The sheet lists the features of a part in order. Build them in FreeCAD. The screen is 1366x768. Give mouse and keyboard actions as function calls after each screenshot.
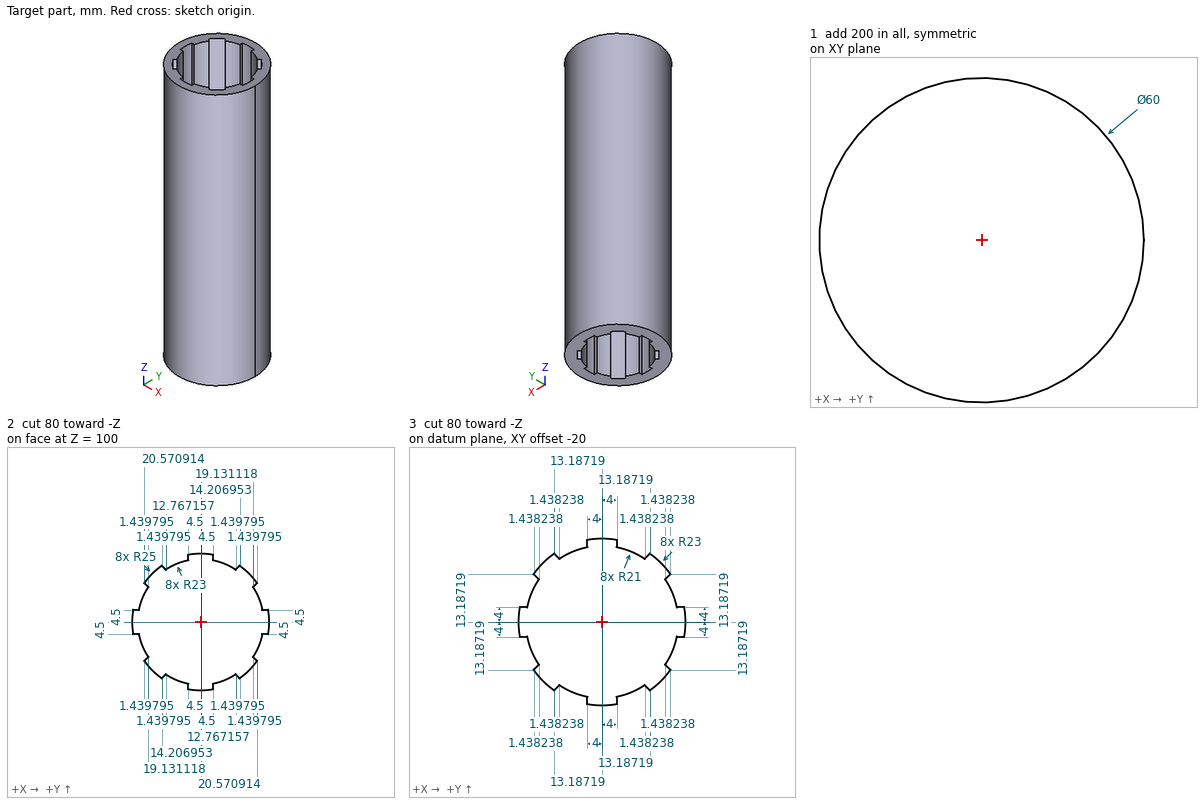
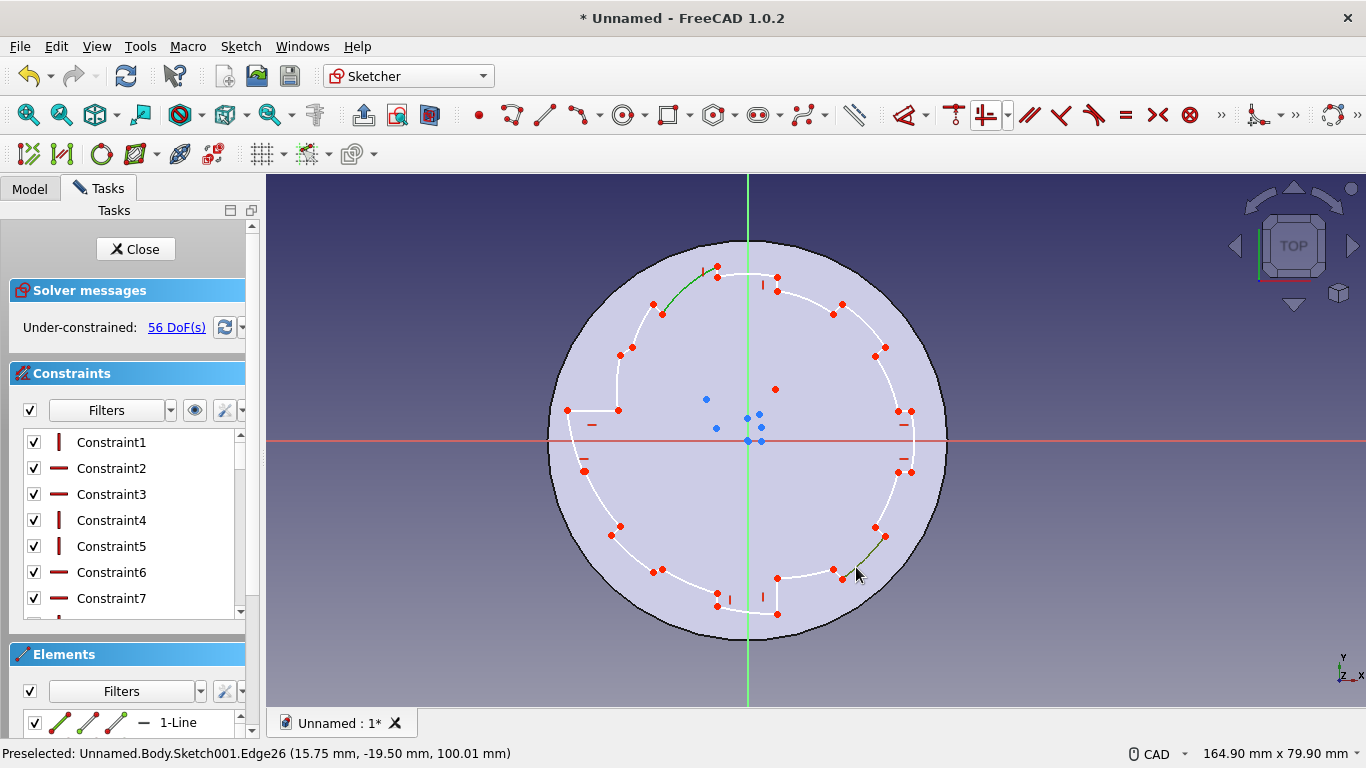
click(954, 116)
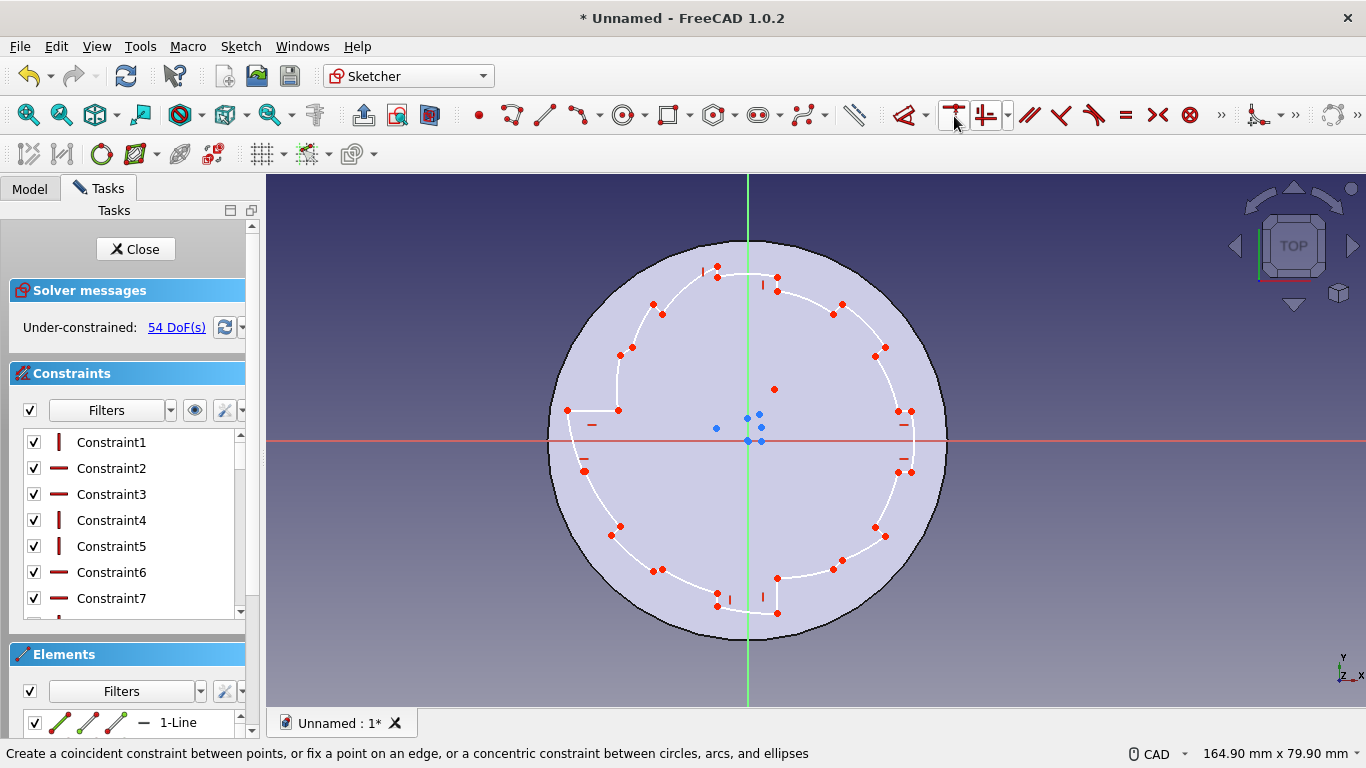
click(698, 278)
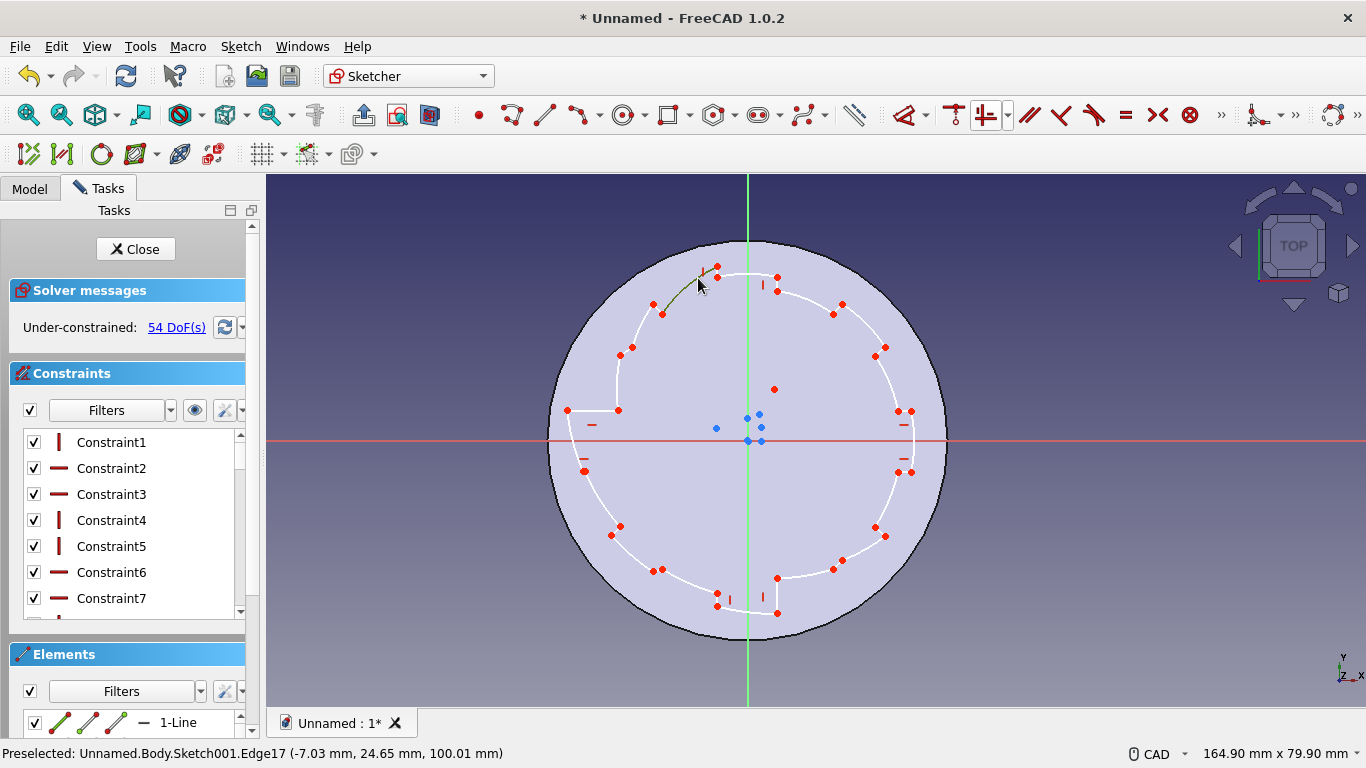
click(884, 511)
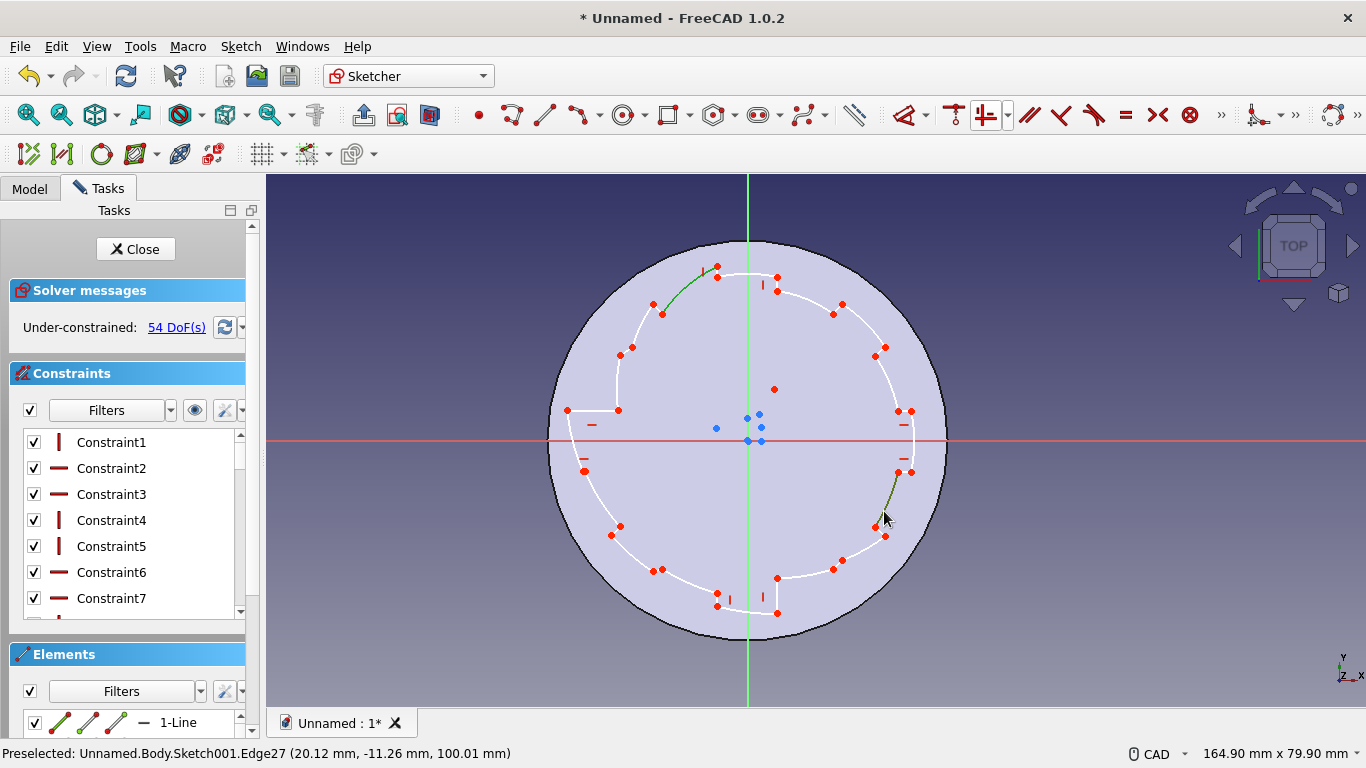
click(954, 116)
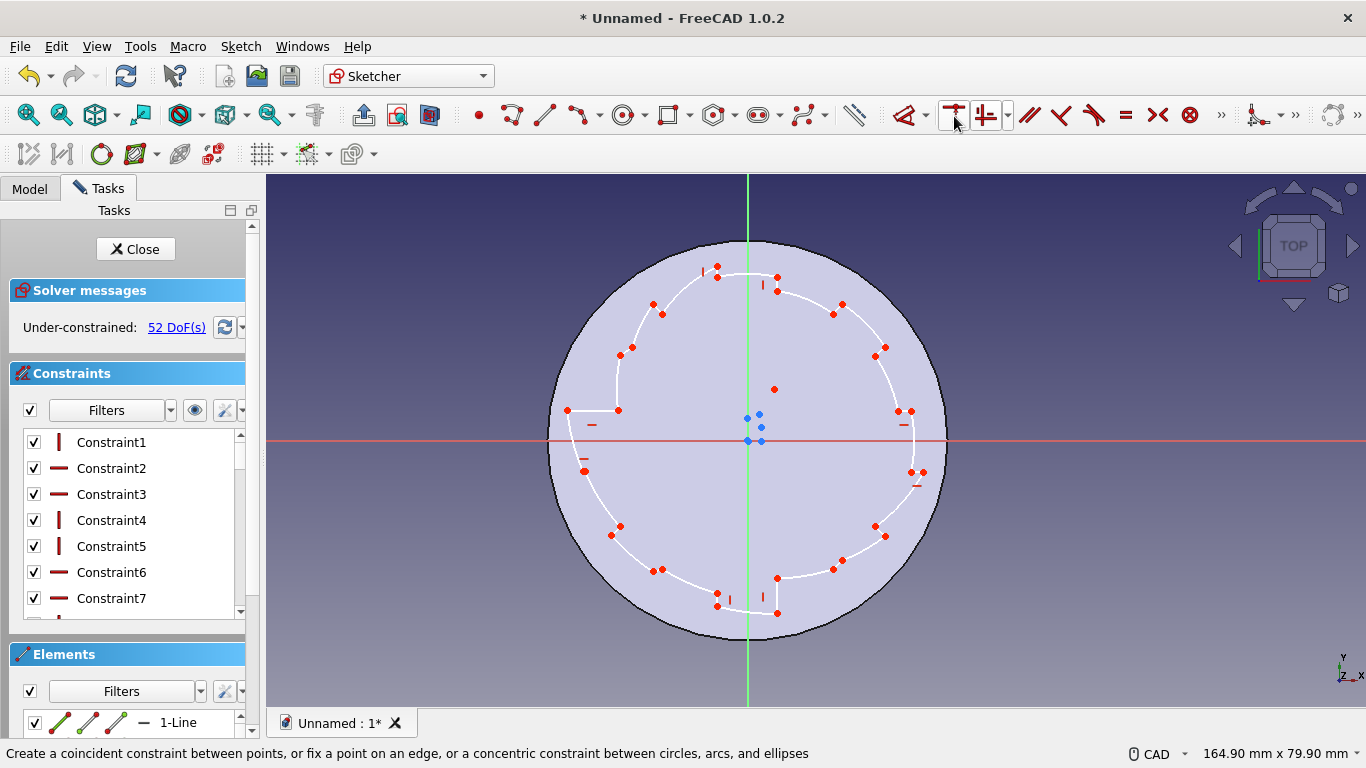
click(698, 278)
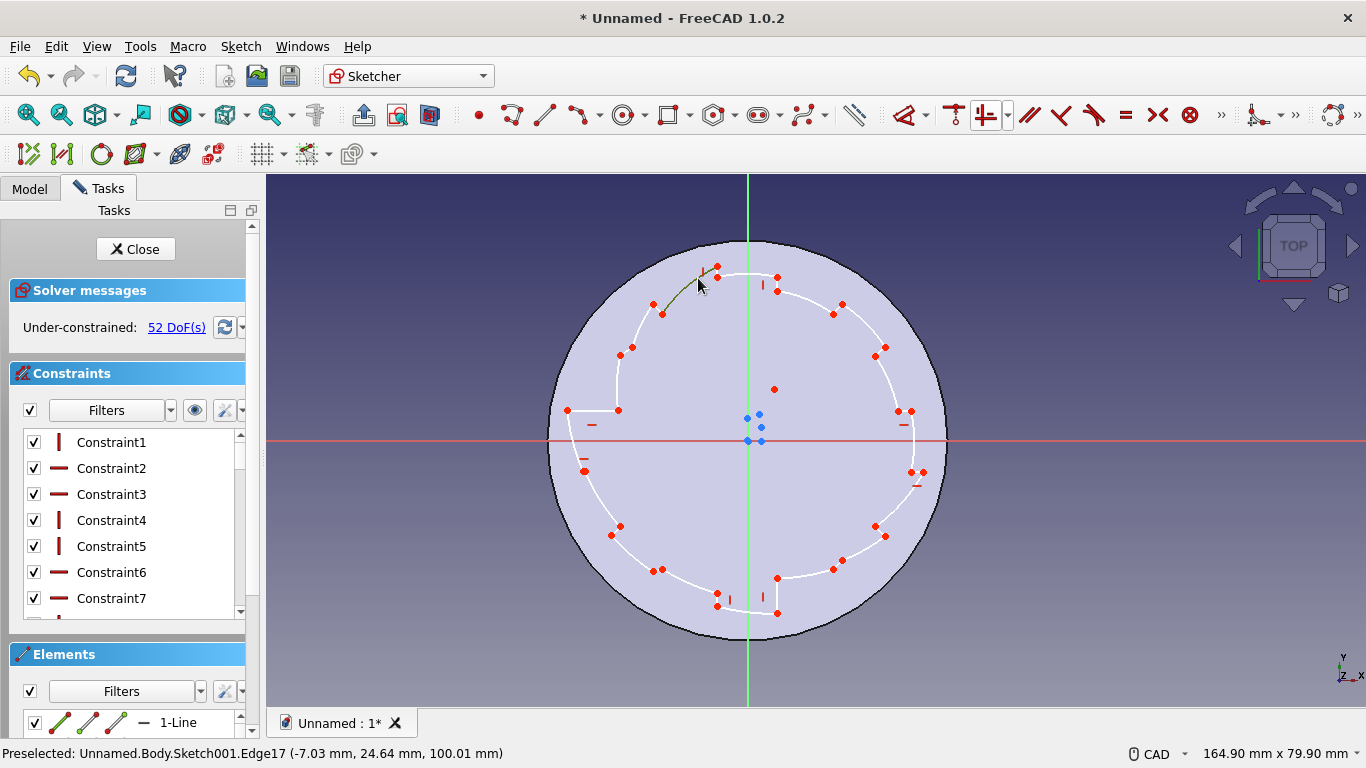
click(914, 454)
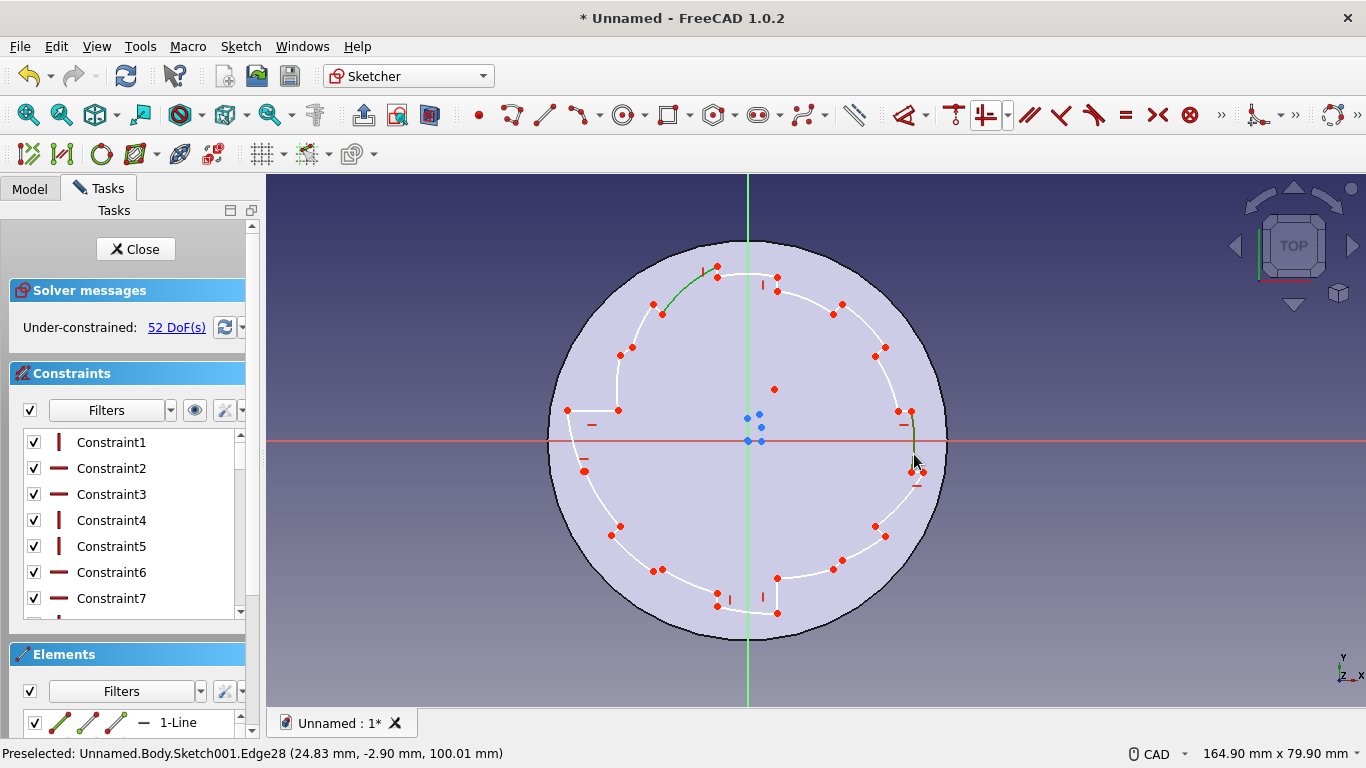
click(954, 116)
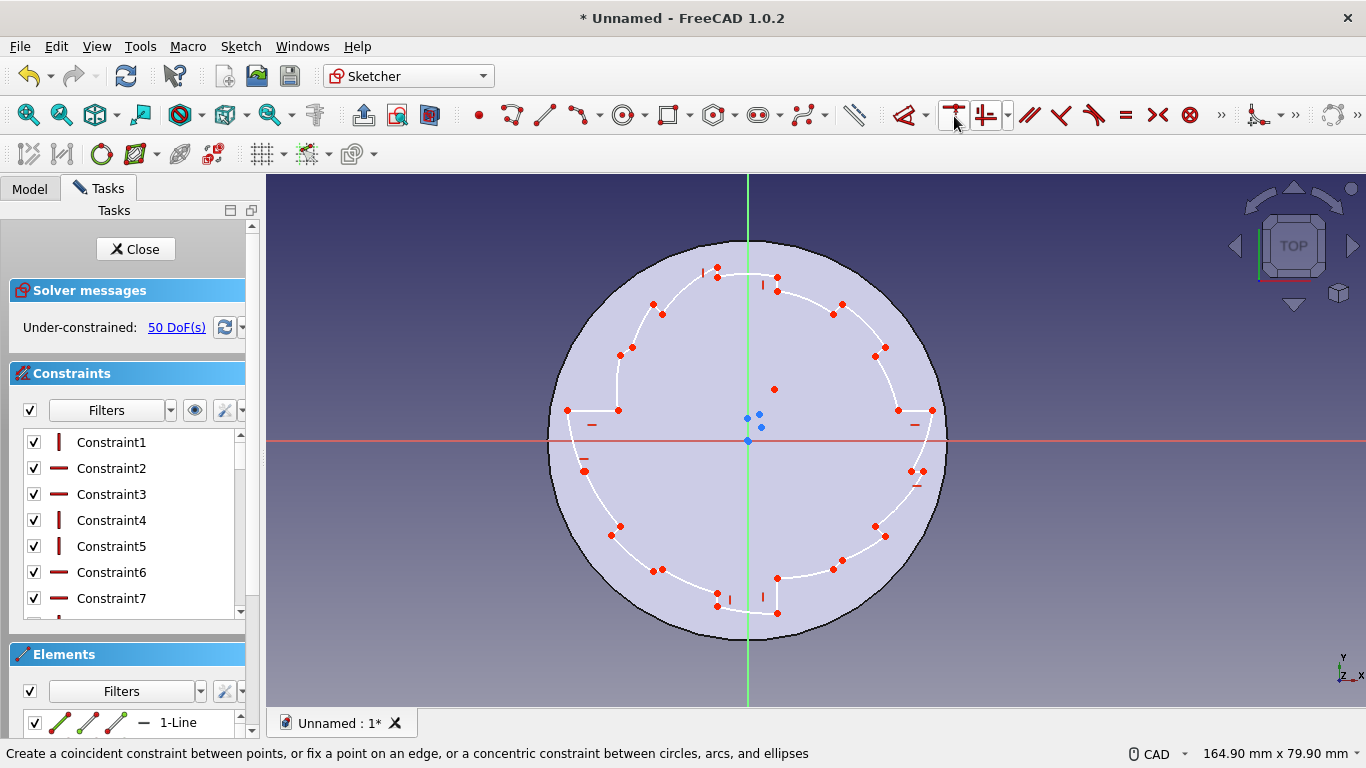
click(698, 278)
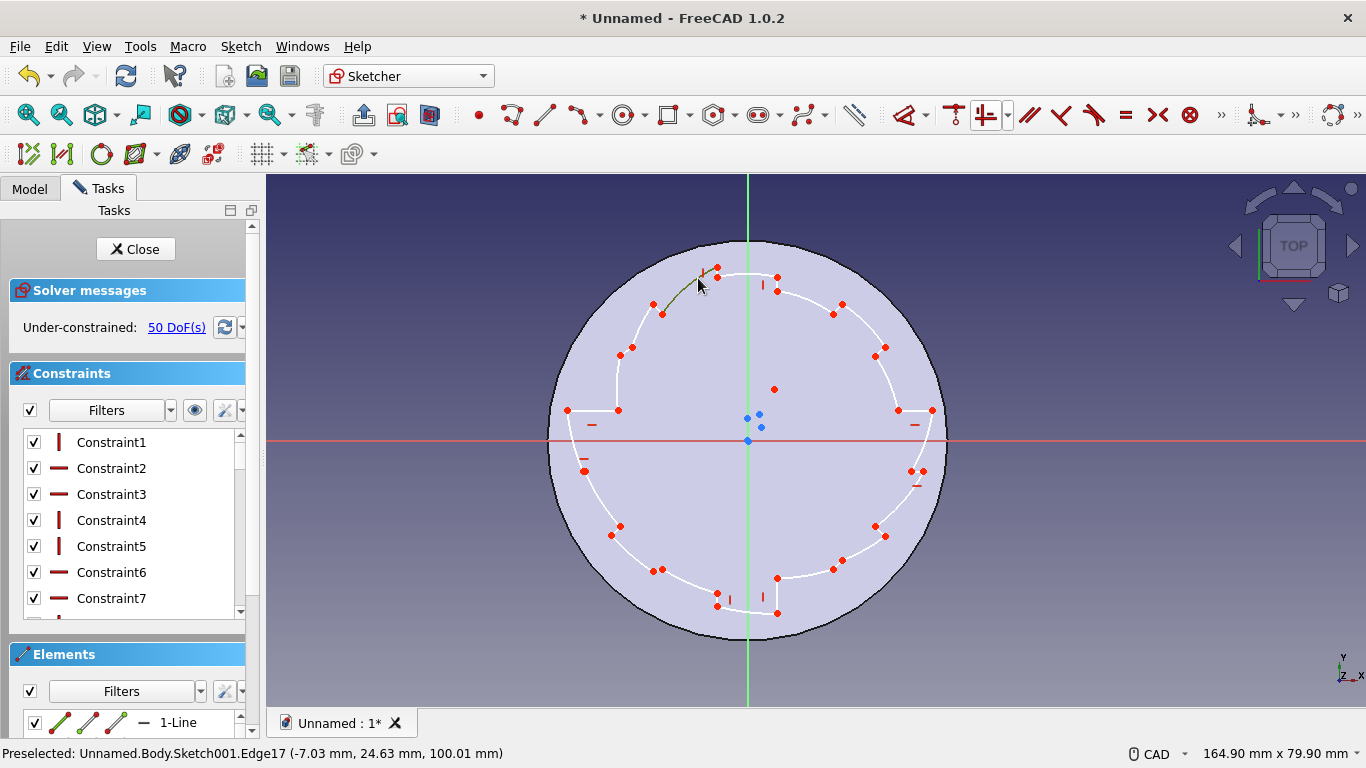
click(894, 394)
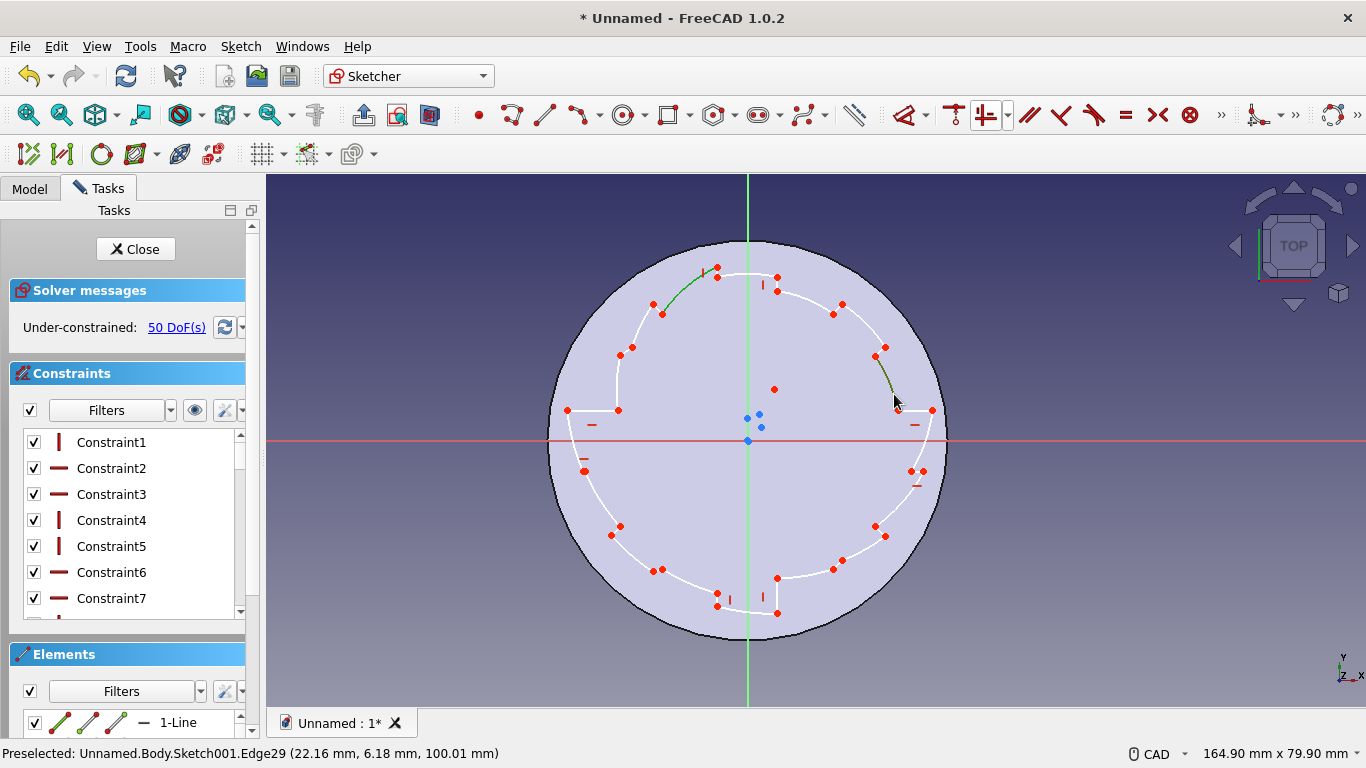
click(954, 116)